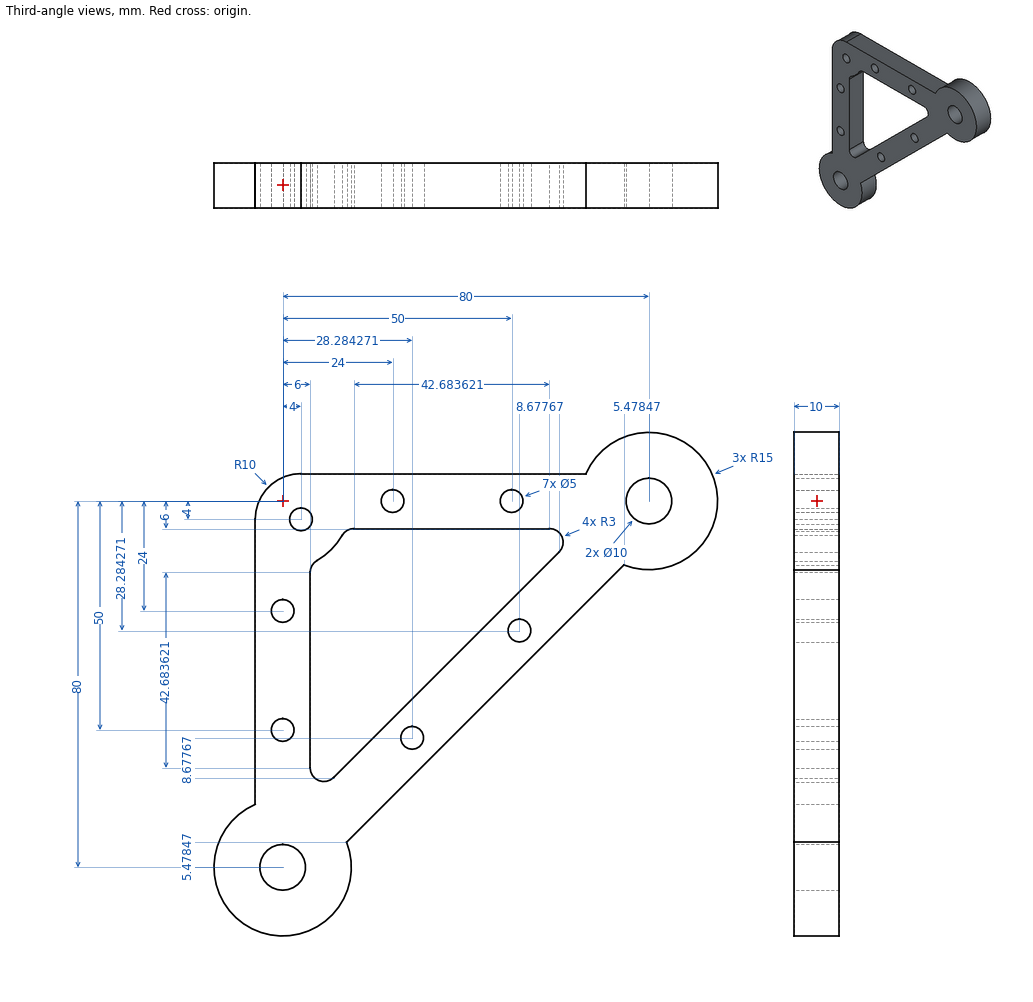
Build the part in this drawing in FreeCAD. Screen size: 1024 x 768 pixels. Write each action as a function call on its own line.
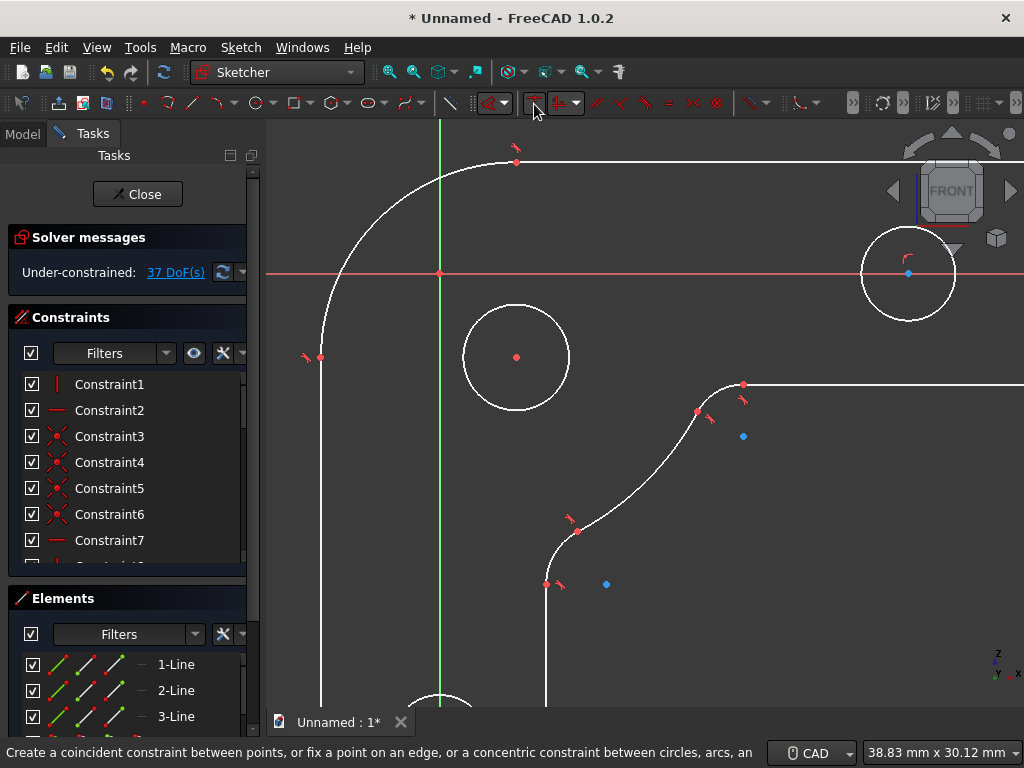
scroll(394, 231, down, 8)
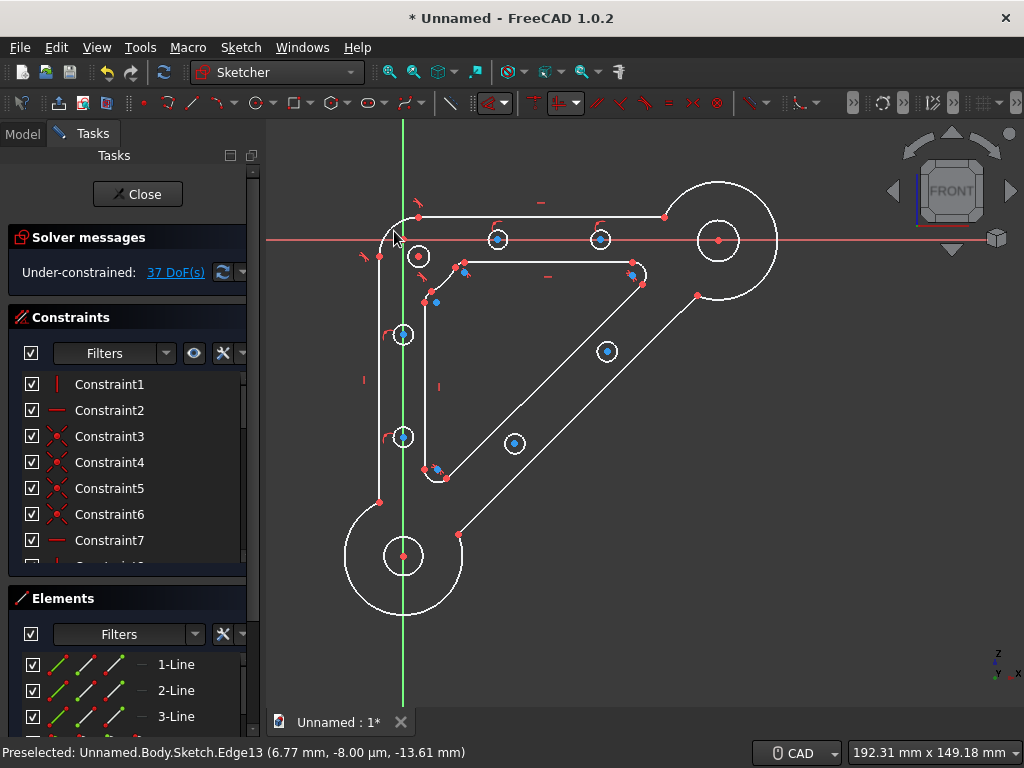
click(769, 271)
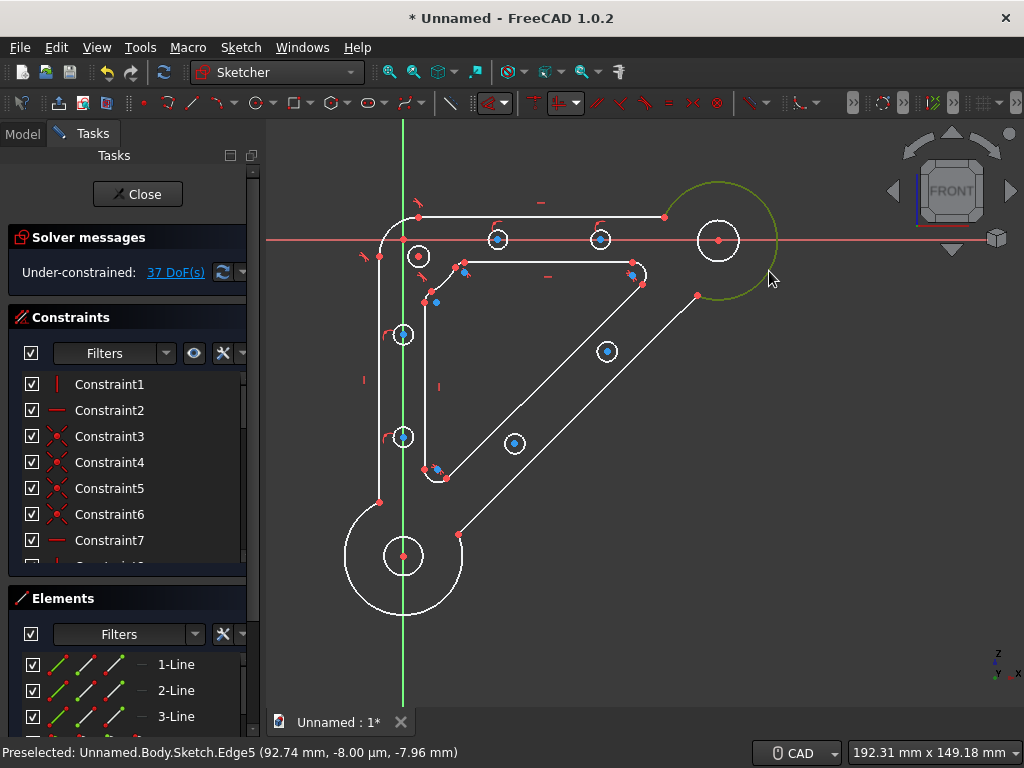
click(346, 571)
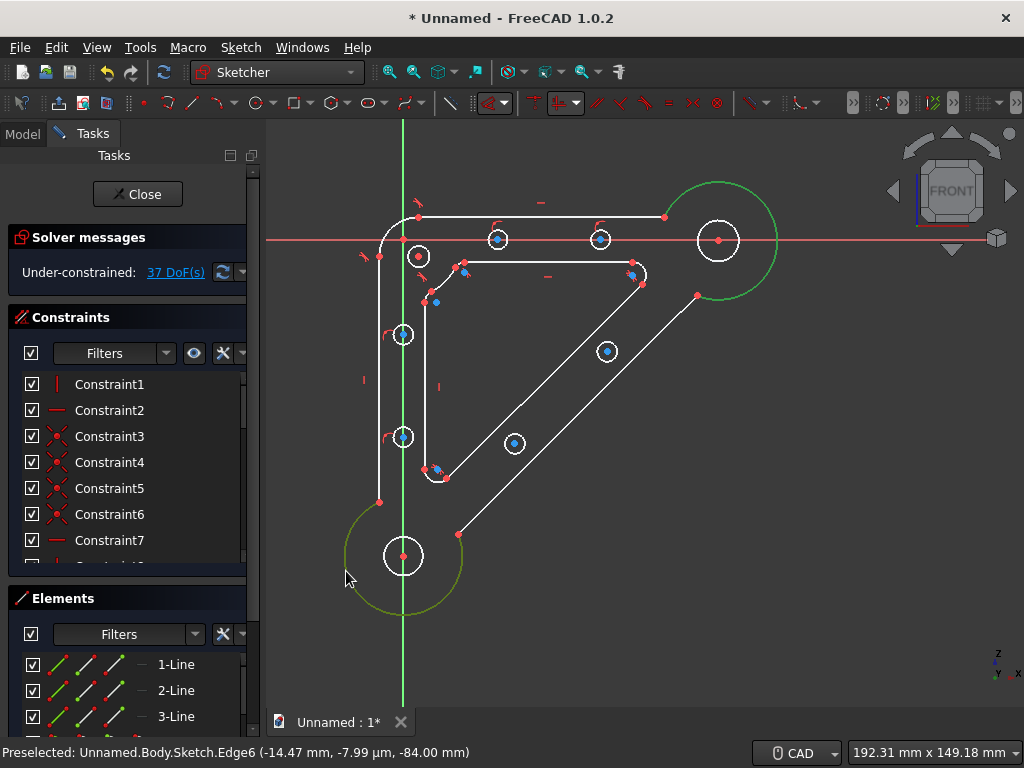
scroll(440, 286, up, 2)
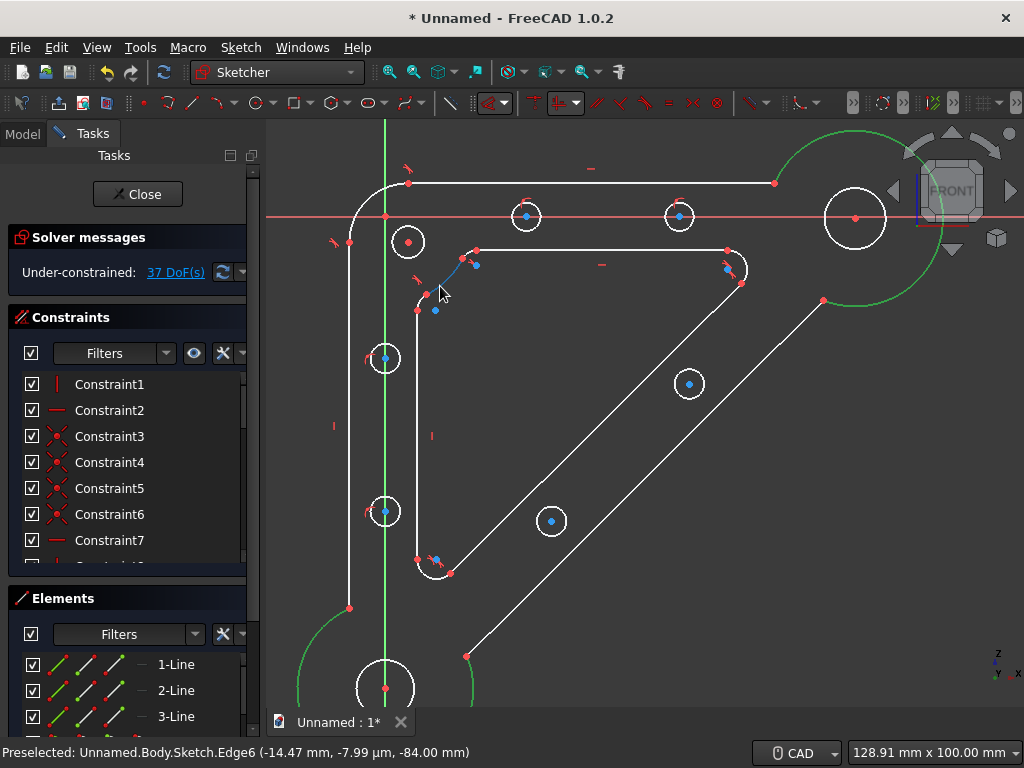
click(440, 286)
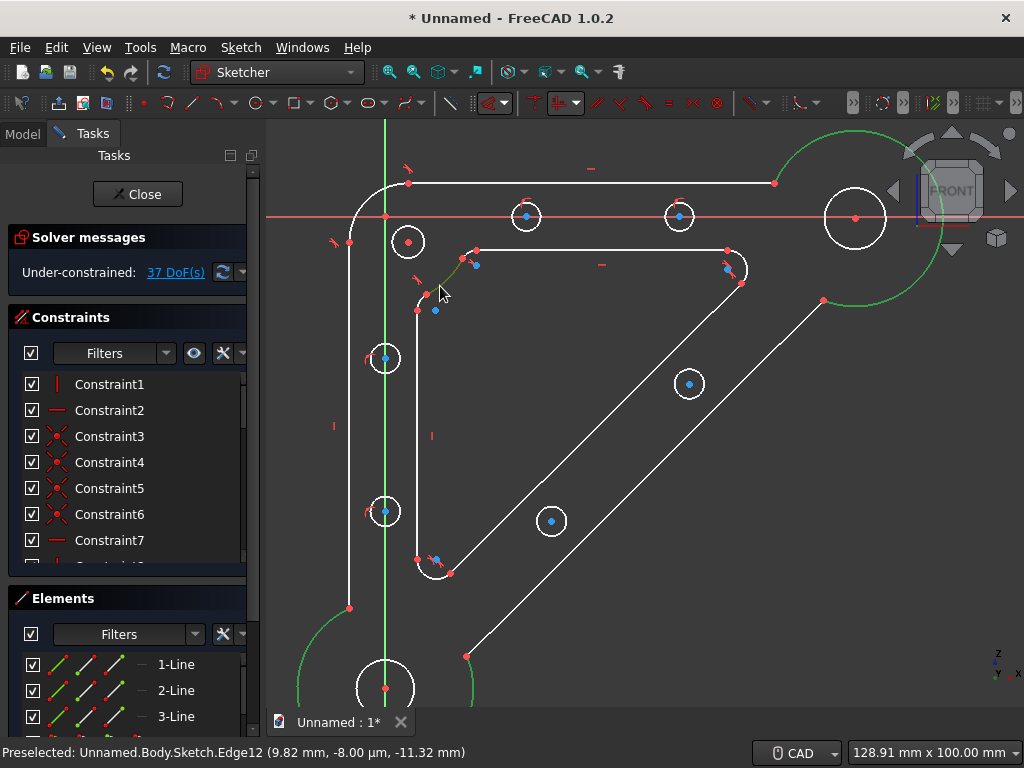
click(670, 104)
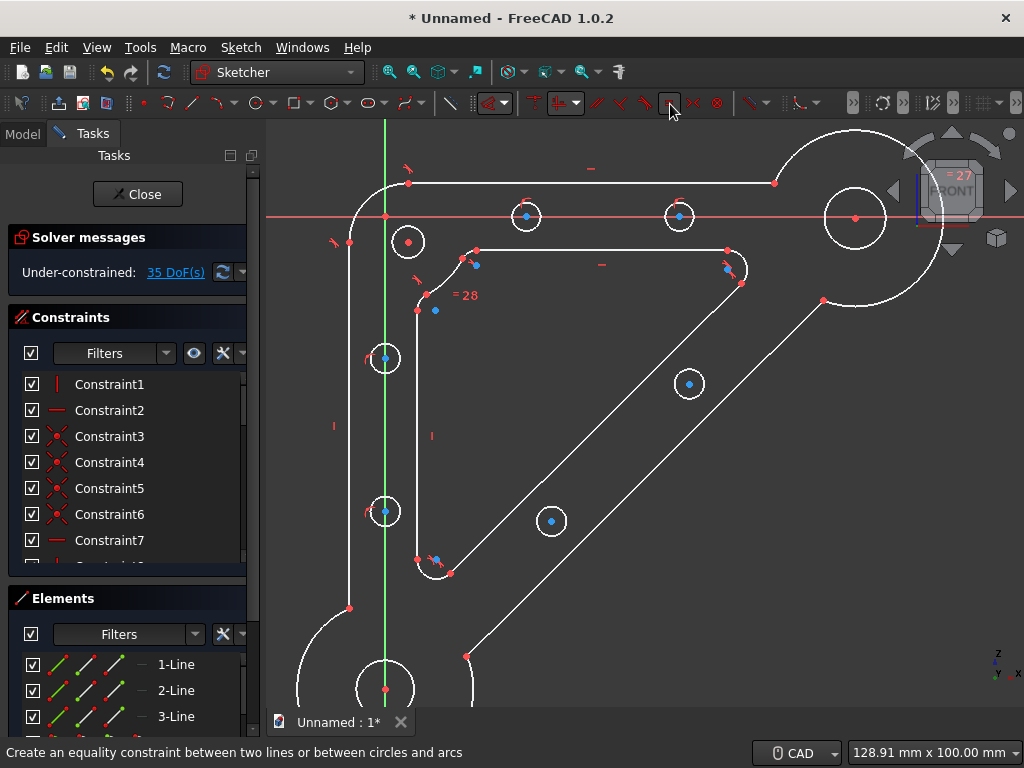
click(747, 271)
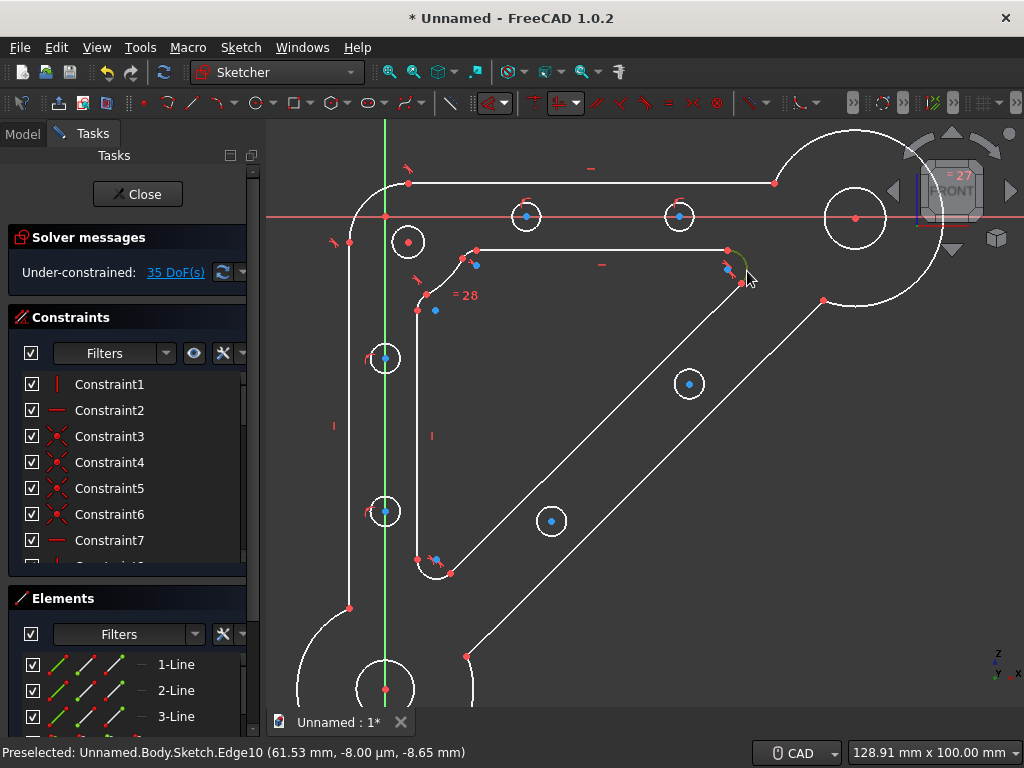
scroll(469, 252, up, 3)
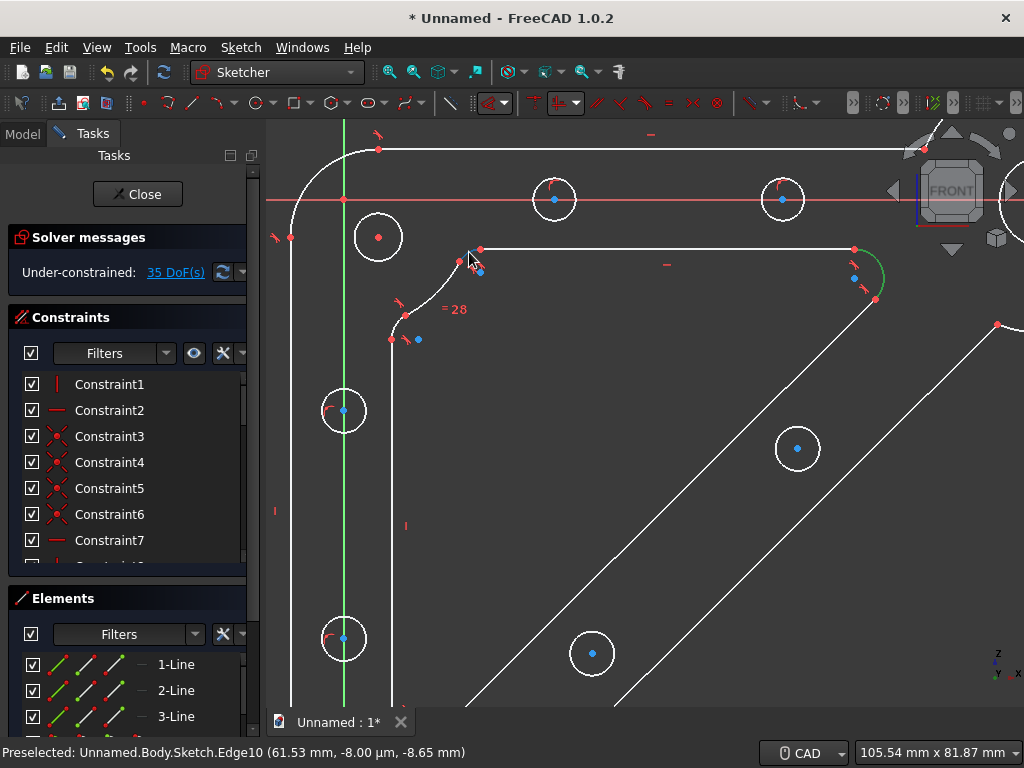
click(468, 253)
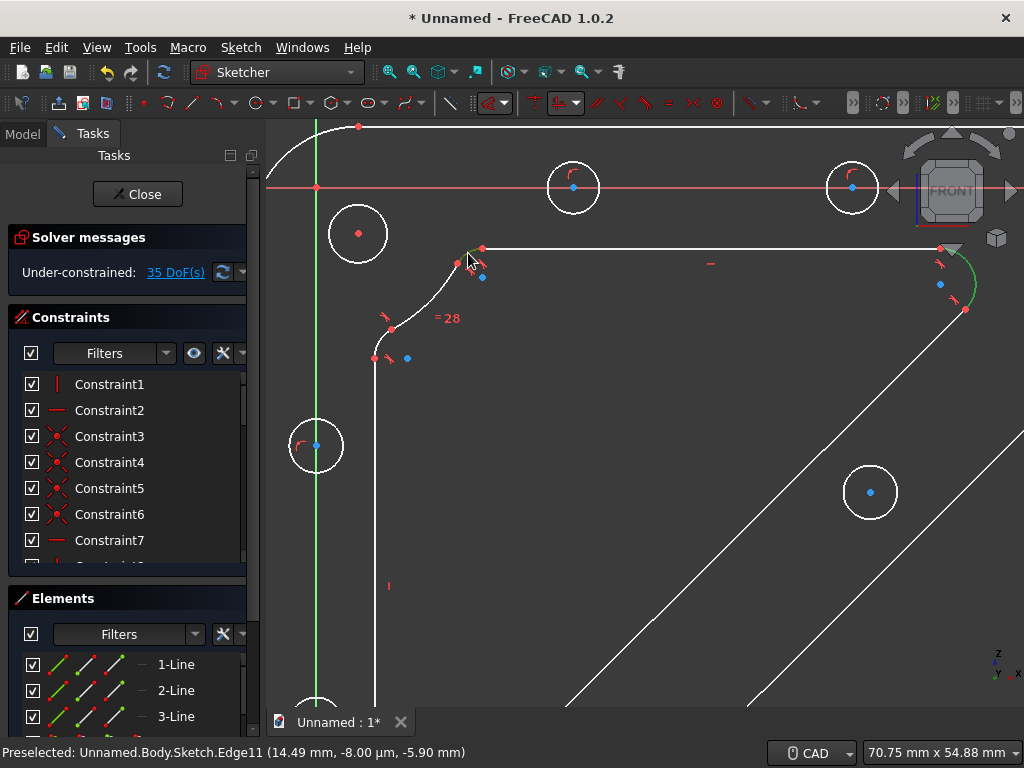
scroll(384, 336, up, 2)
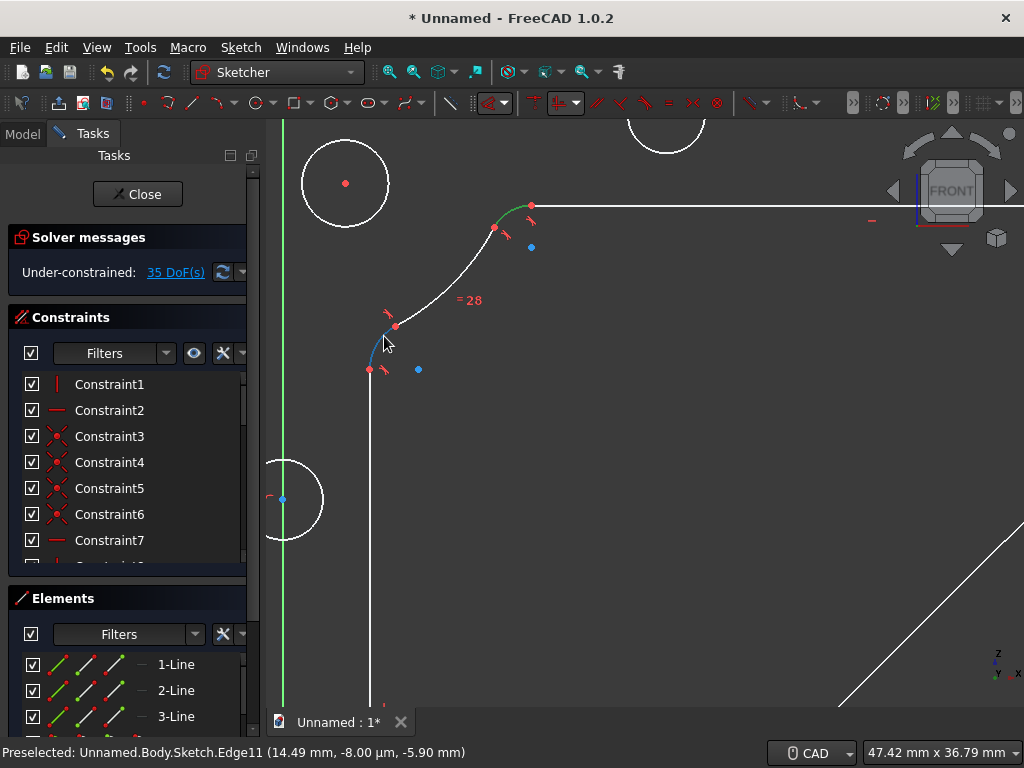
click(383, 336)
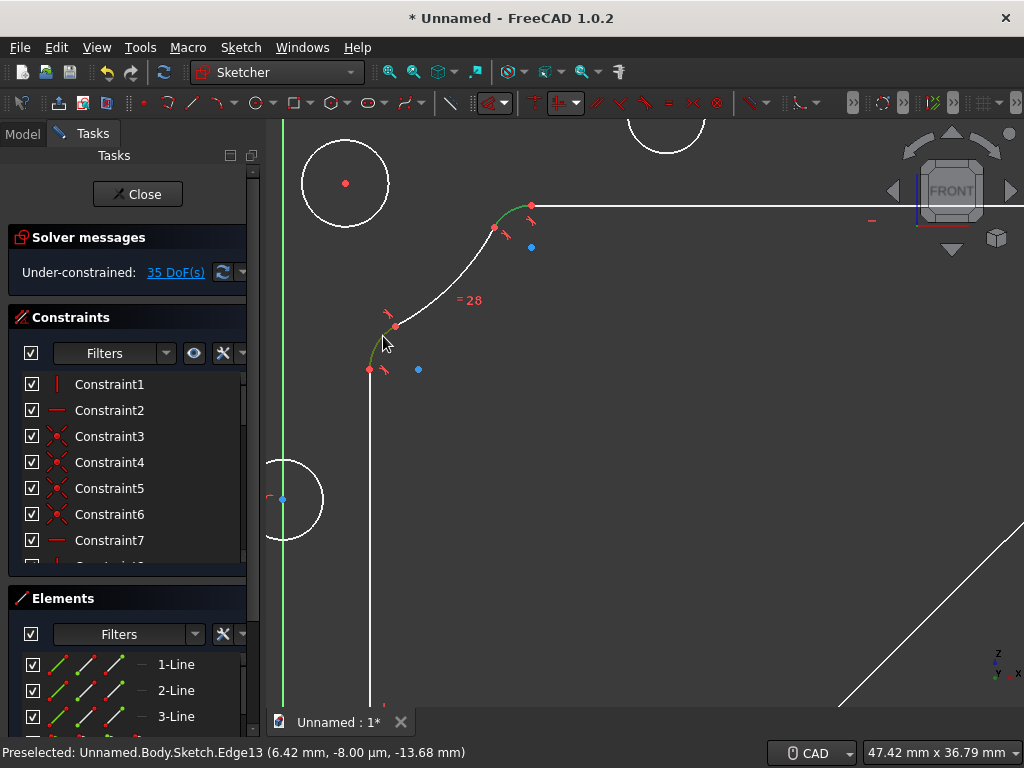
scroll(443, 281, down, 7)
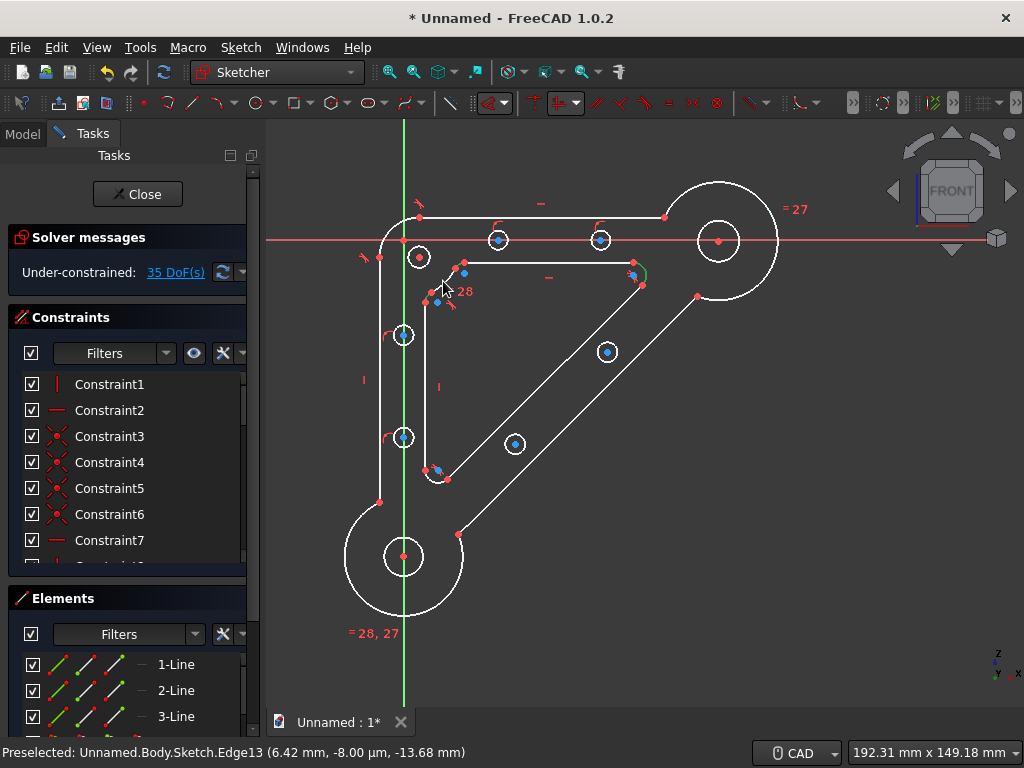
scroll(428, 478, up, 3)